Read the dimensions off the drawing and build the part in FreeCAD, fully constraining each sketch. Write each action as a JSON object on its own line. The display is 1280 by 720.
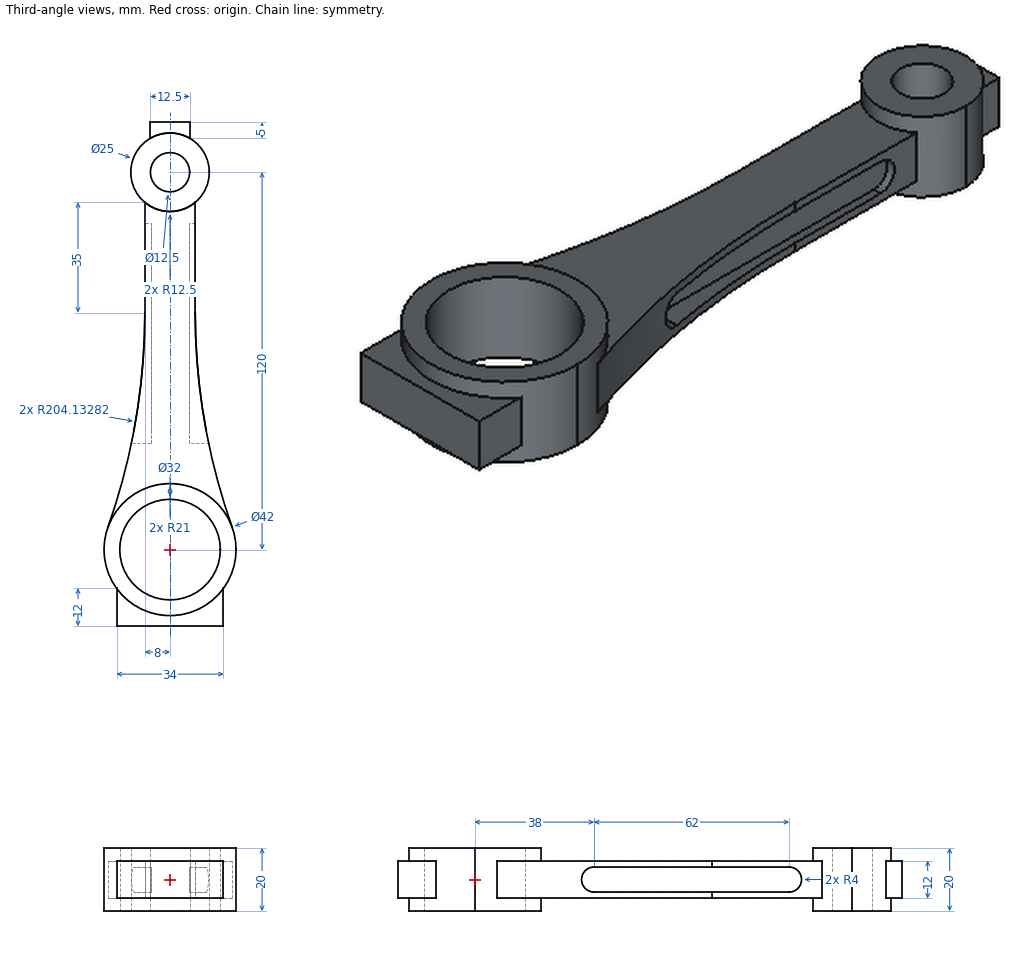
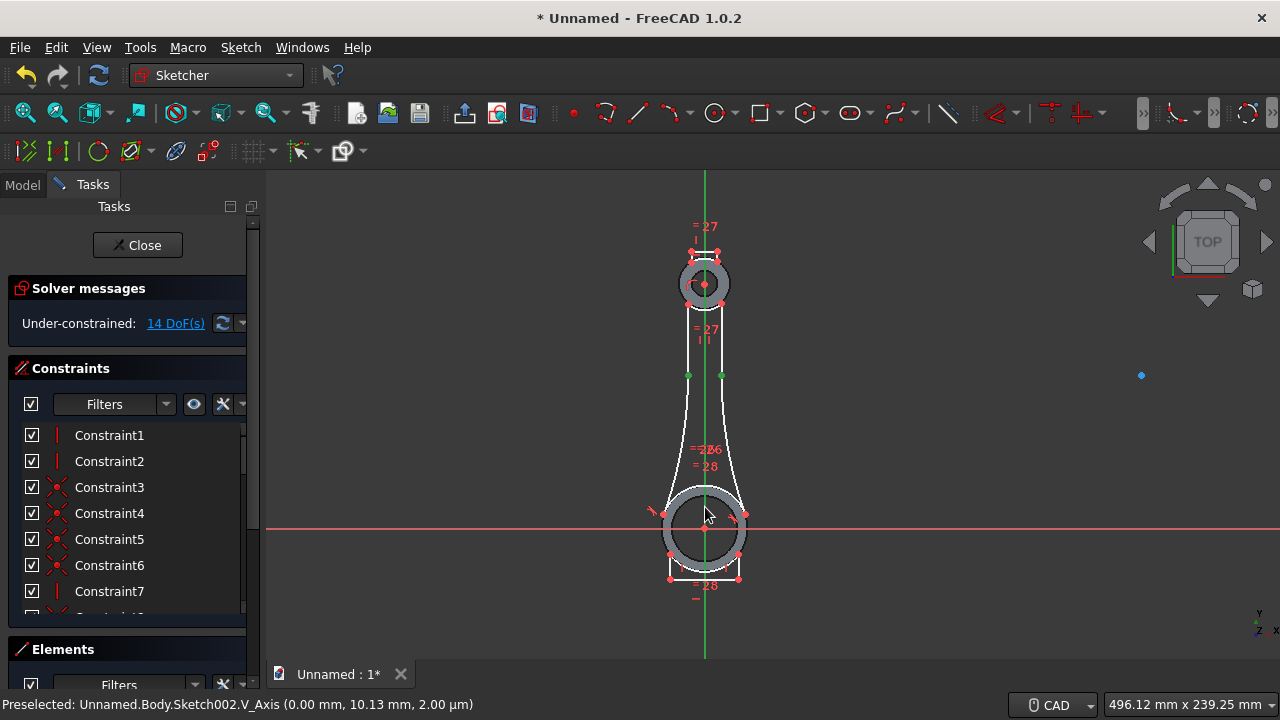
{"action": "key", "text": "s"}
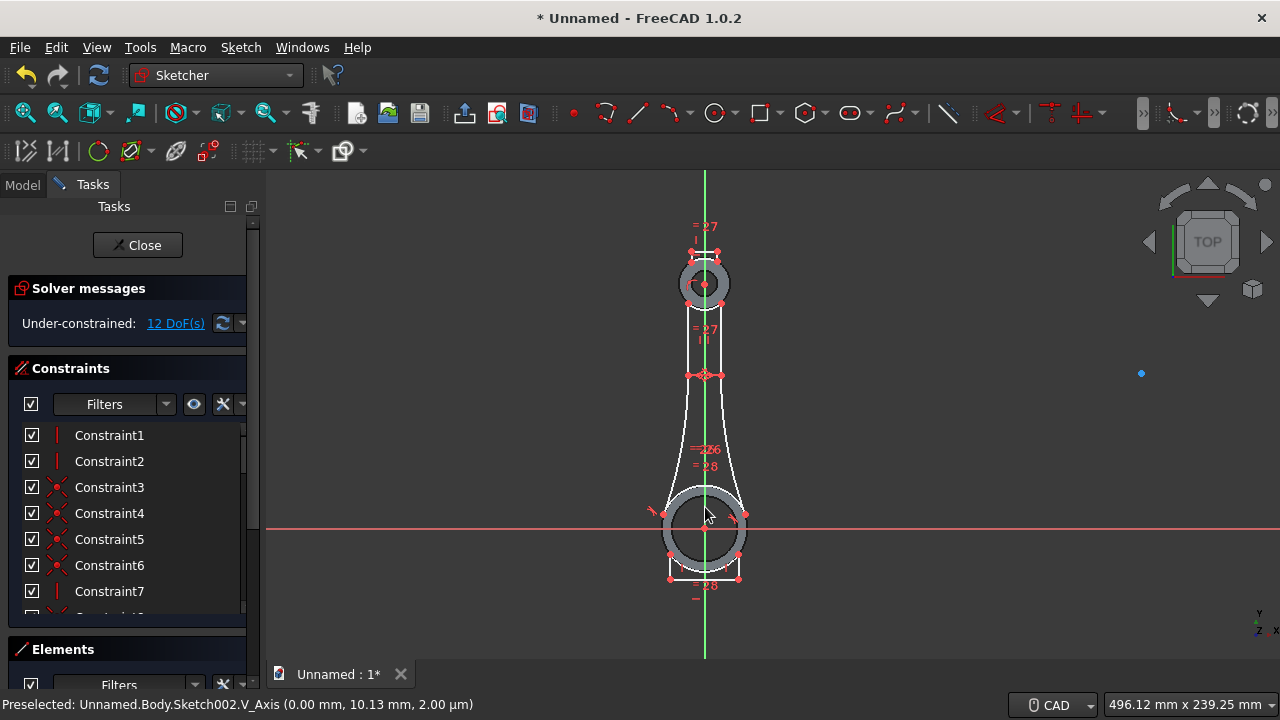
{"action": "left_click", "coordinate": [996, 114]}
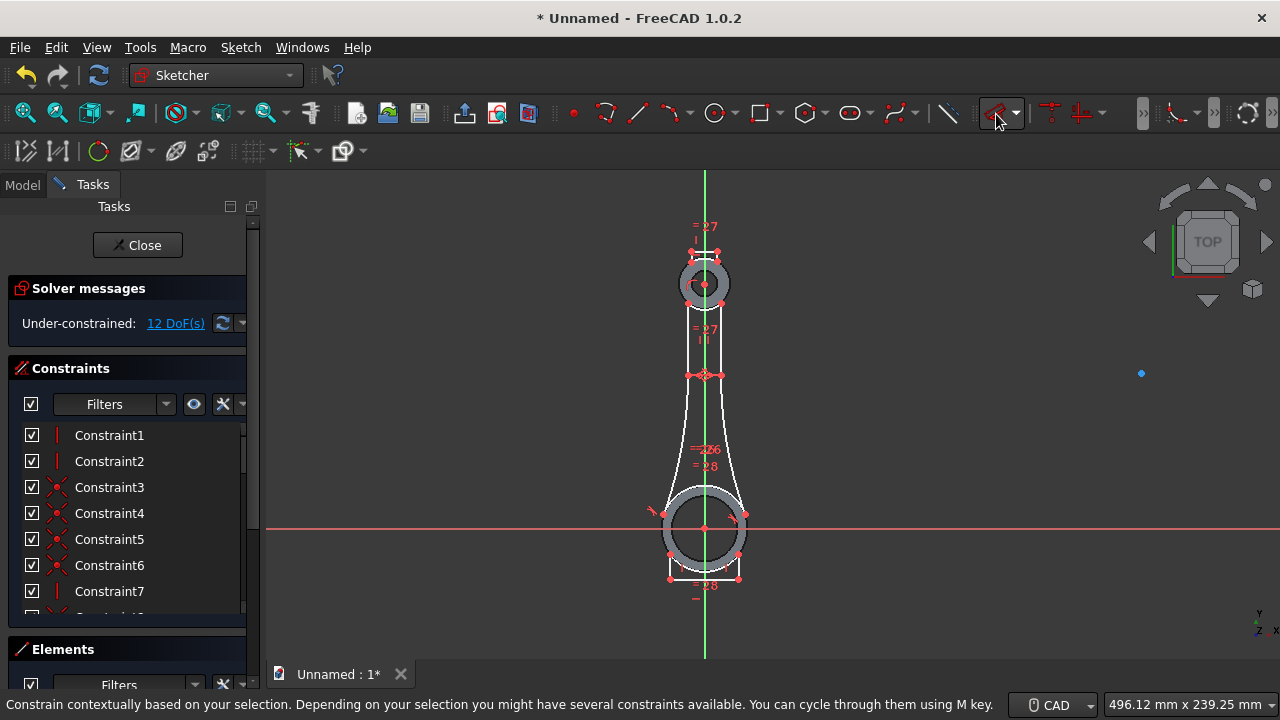
{"action": "left_click", "coordinate": [676, 474]}
{"action": "left_click", "coordinate": [754, 493]}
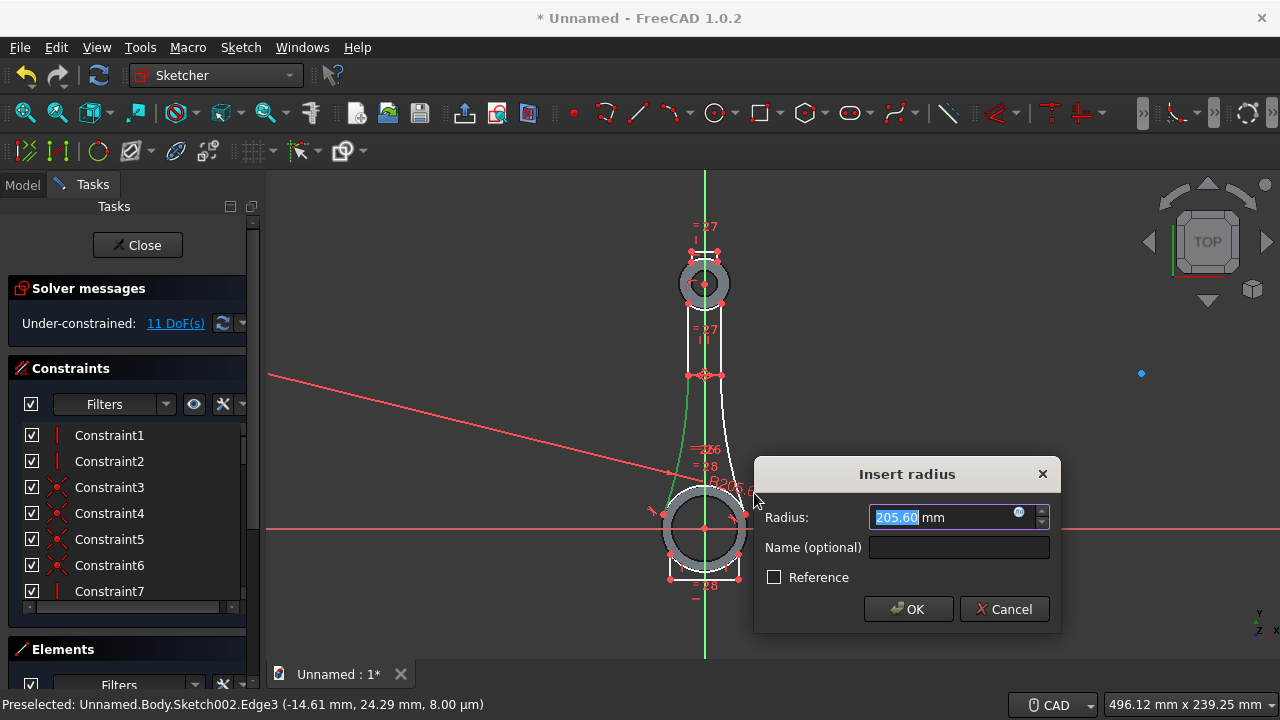
{"action": "type", "text": "204.13282"}
{"action": "key", "text": "Return"}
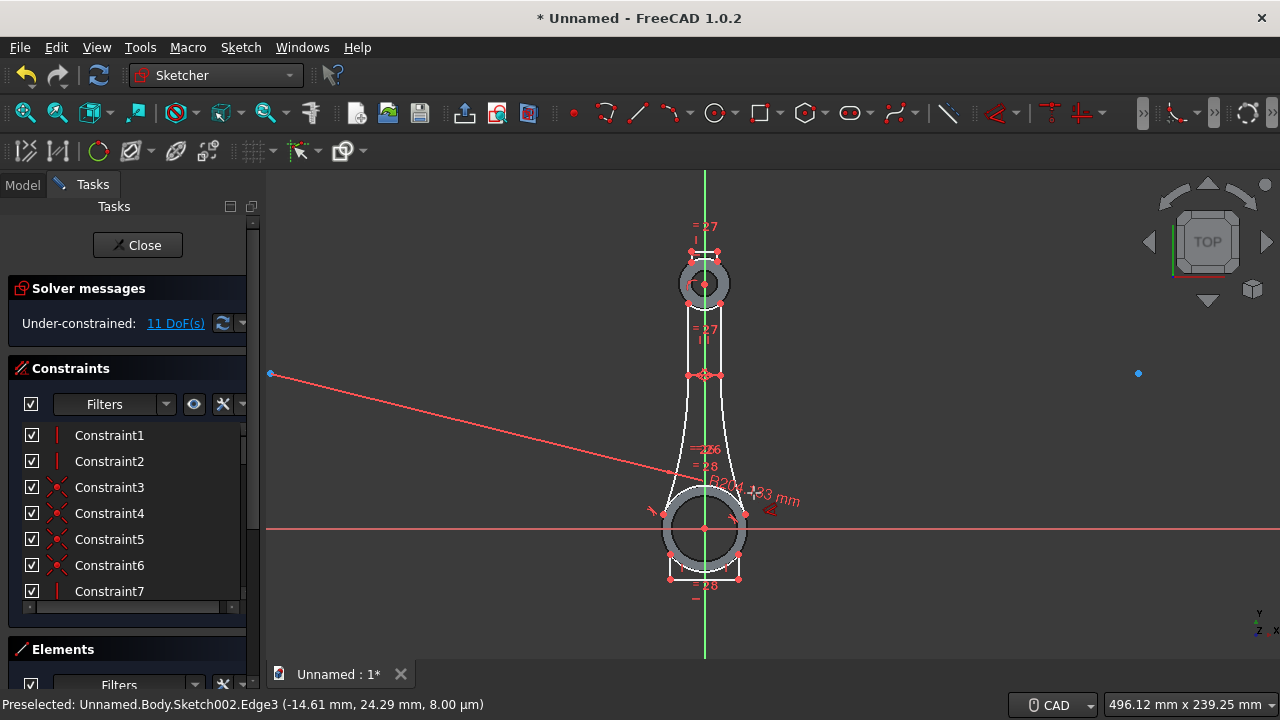
{"action": "left_click", "coordinate": [725, 491]}
{"action": "left_click", "coordinate": [770, 564]}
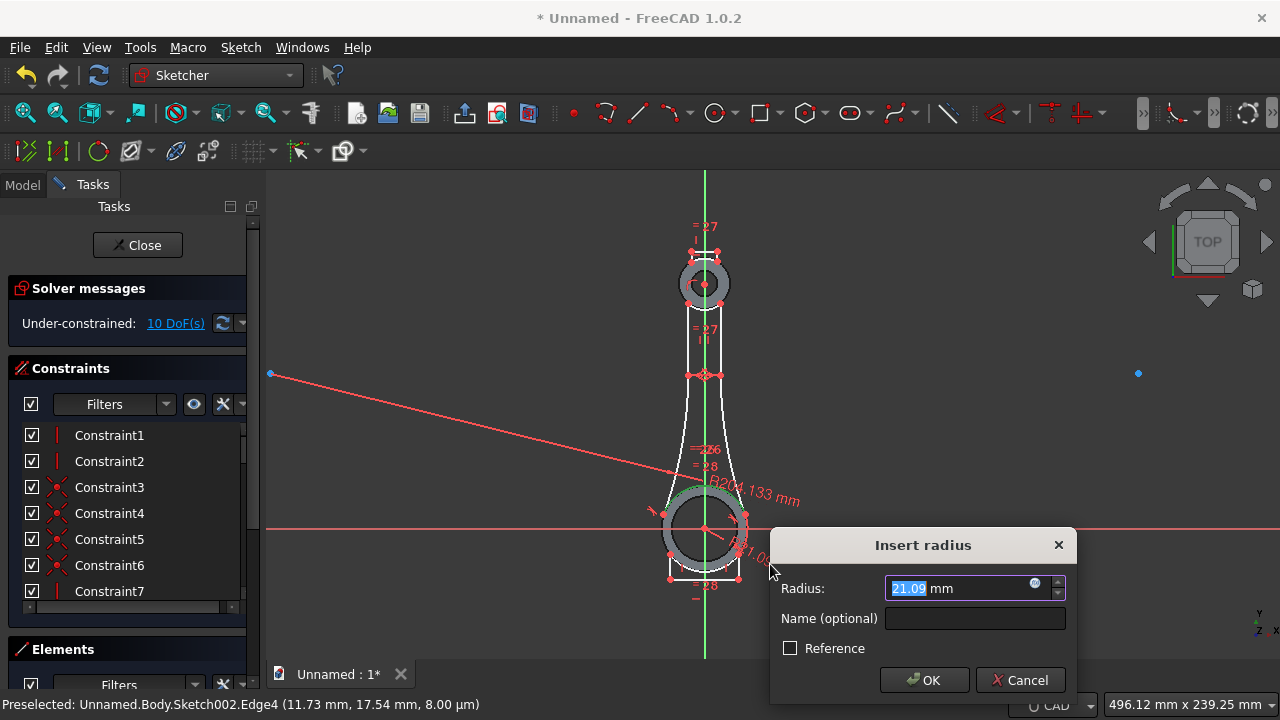
{"action": "type", "text": "21"}
{"action": "key", "text": "Return"}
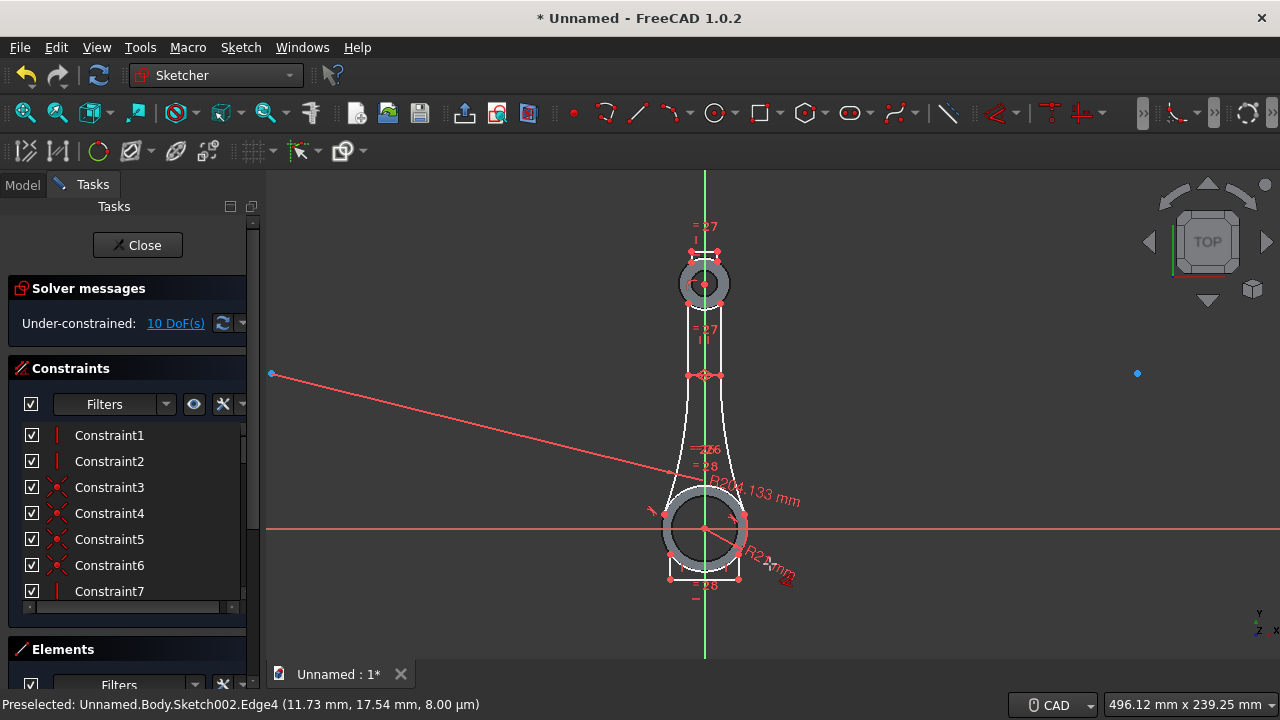
{"action": "scroll", "coordinate": [705, 310], "scroll_direction": "up", "scroll_amount": 3}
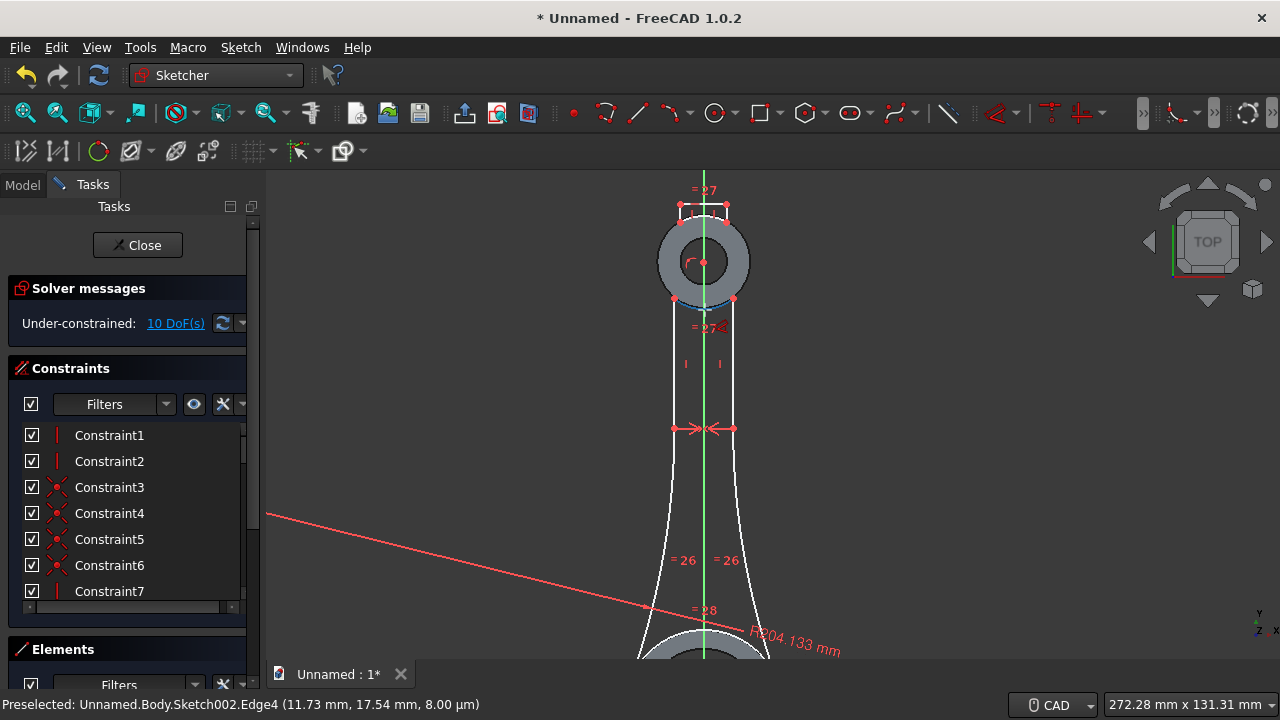
{"action": "left_click", "coordinate": [704, 309]}
{"action": "left_click", "coordinate": [638, 305]}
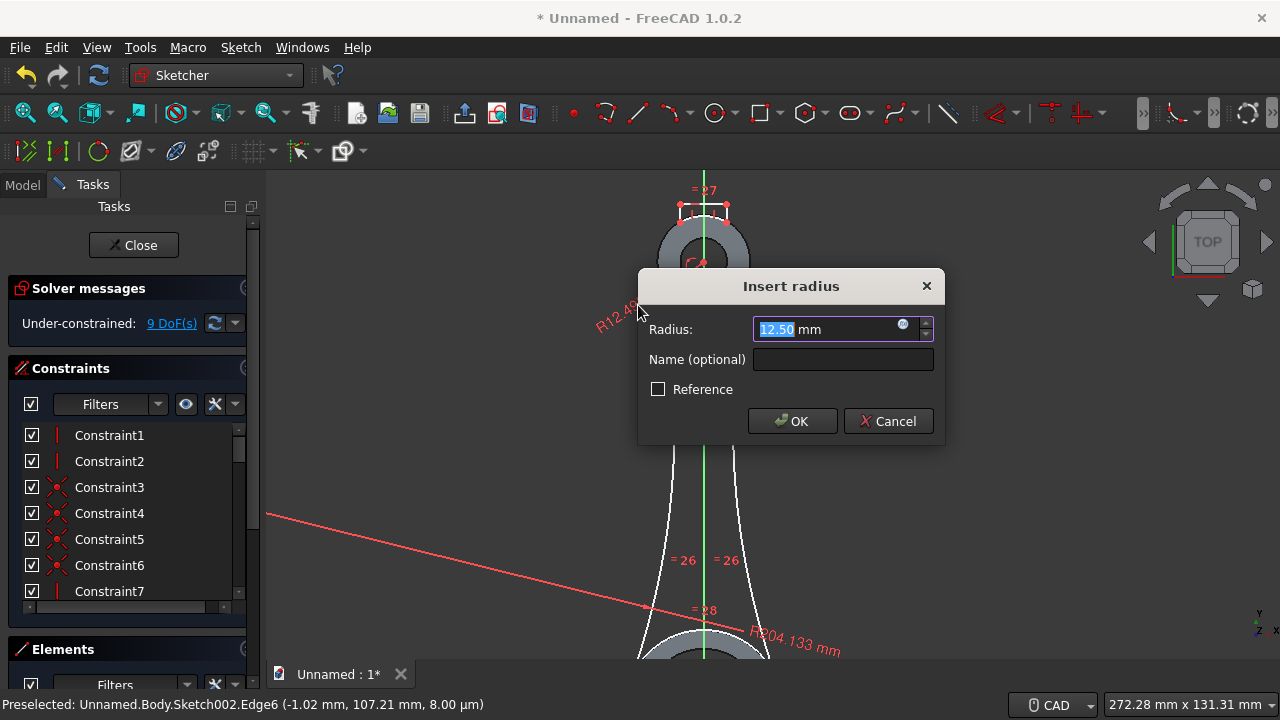
{"action": "type", "text": "12.5"}
{"action": "key", "text": "Return"}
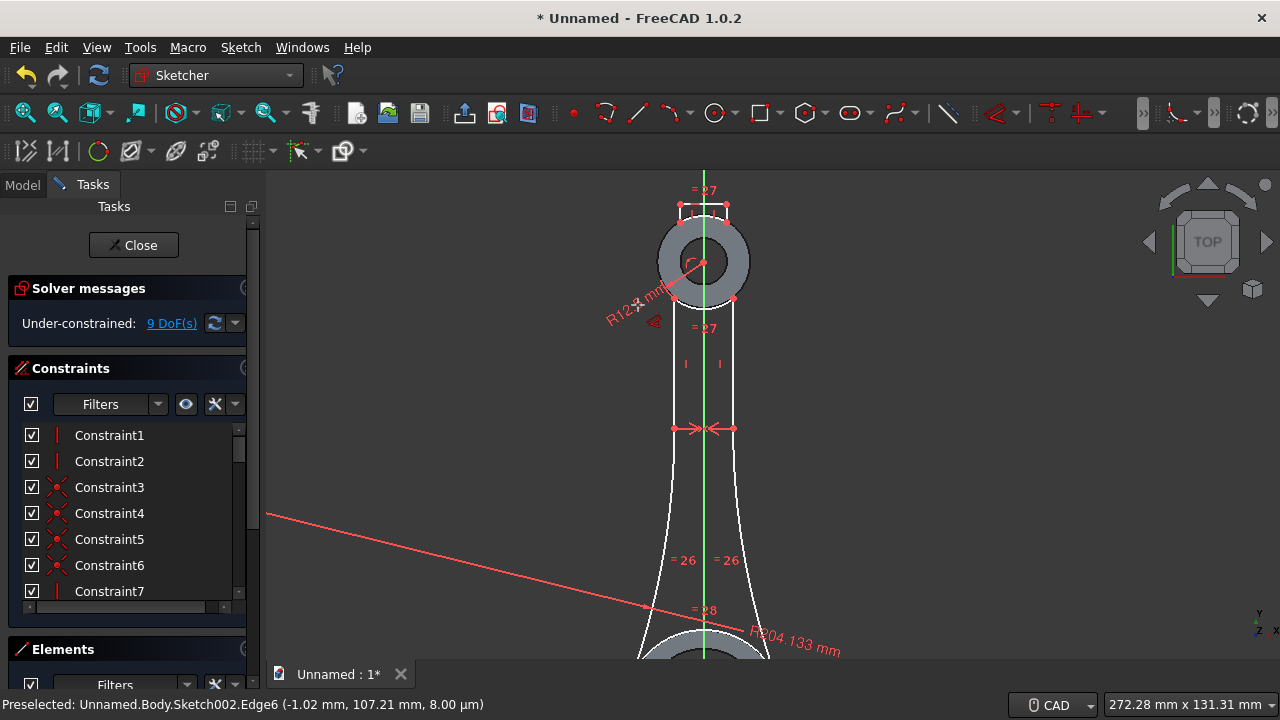
{"action": "scroll", "coordinate": [727, 213], "scroll_direction": "up", "scroll_amount": 4}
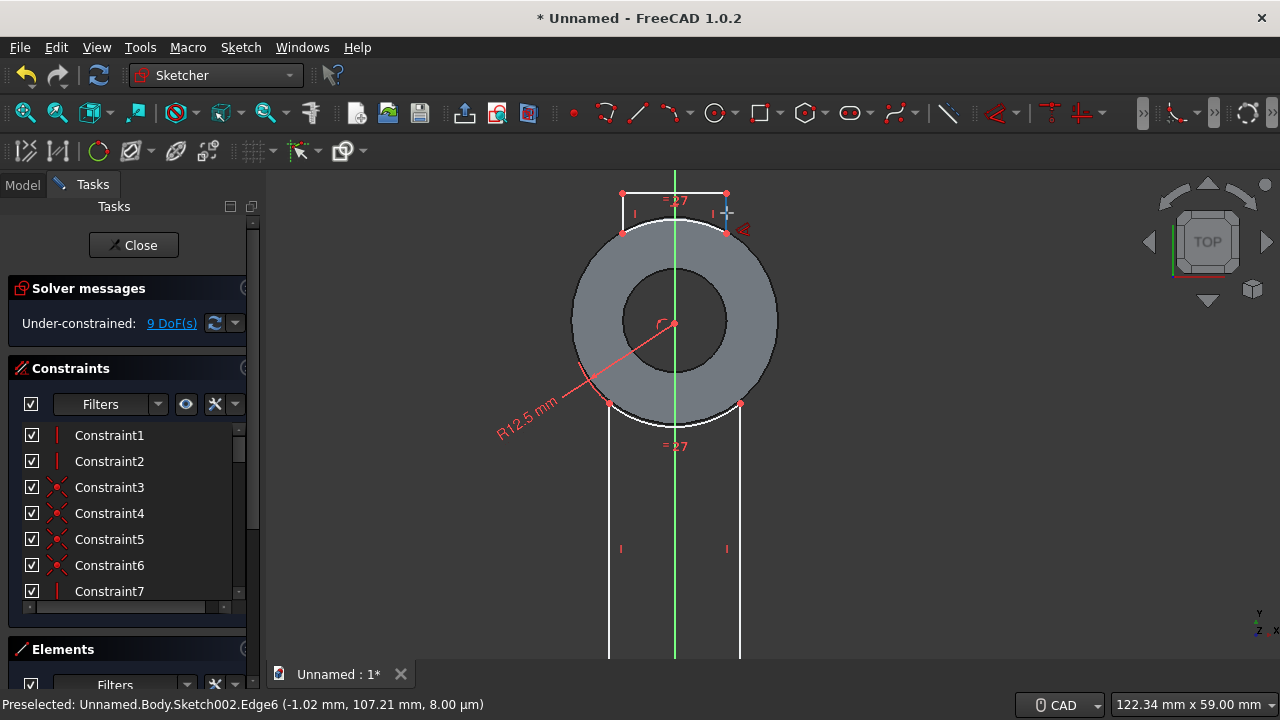
{"action": "left_click", "coordinate": [726, 213]}
{"action": "left_click", "coordinate": [760, 216]}